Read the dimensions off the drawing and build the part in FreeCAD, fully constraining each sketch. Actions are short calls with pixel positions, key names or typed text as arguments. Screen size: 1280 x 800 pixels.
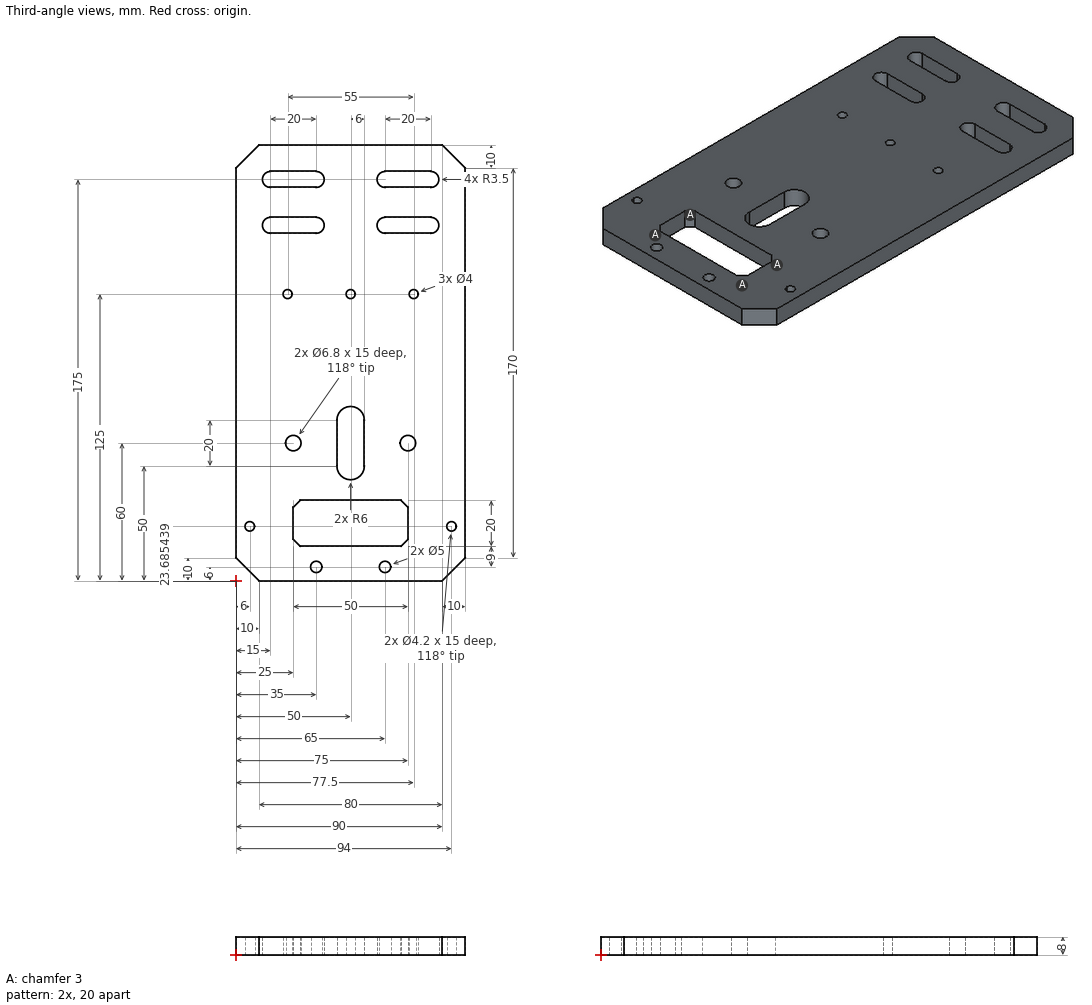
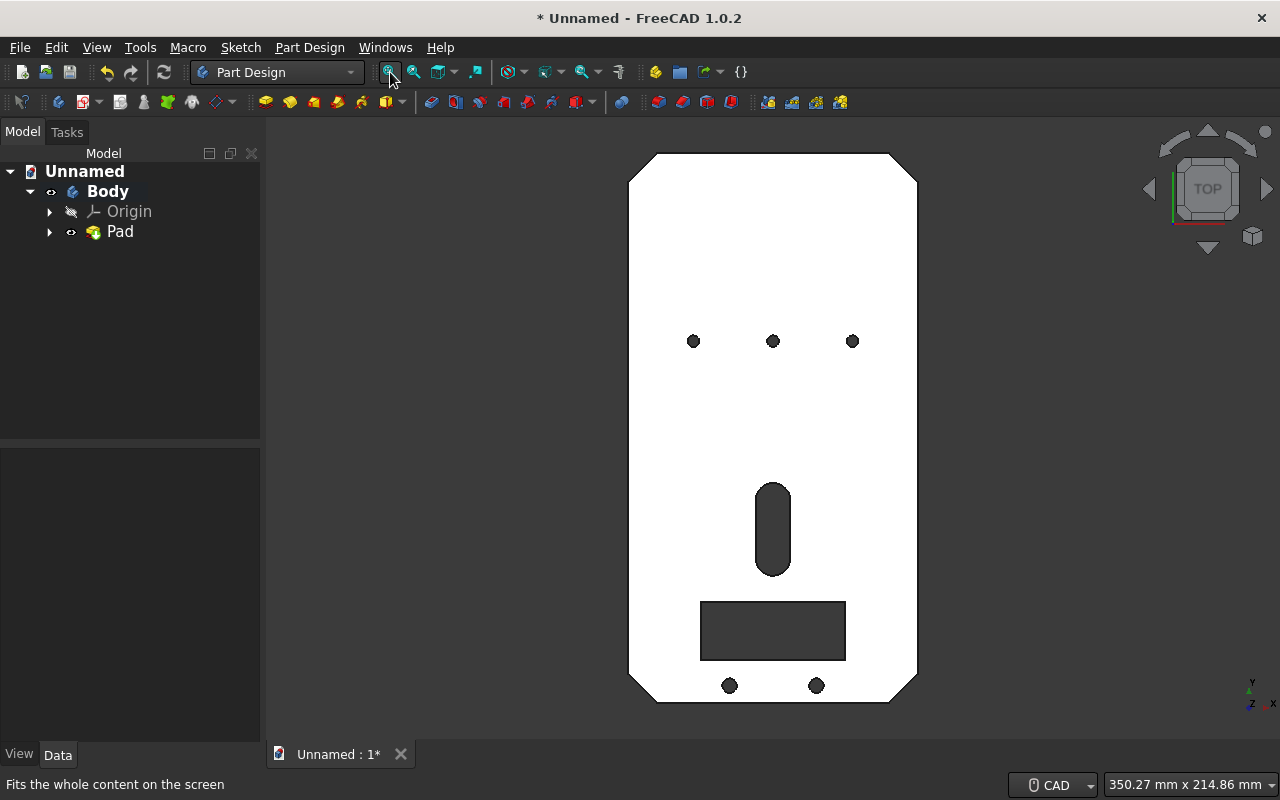
key(1)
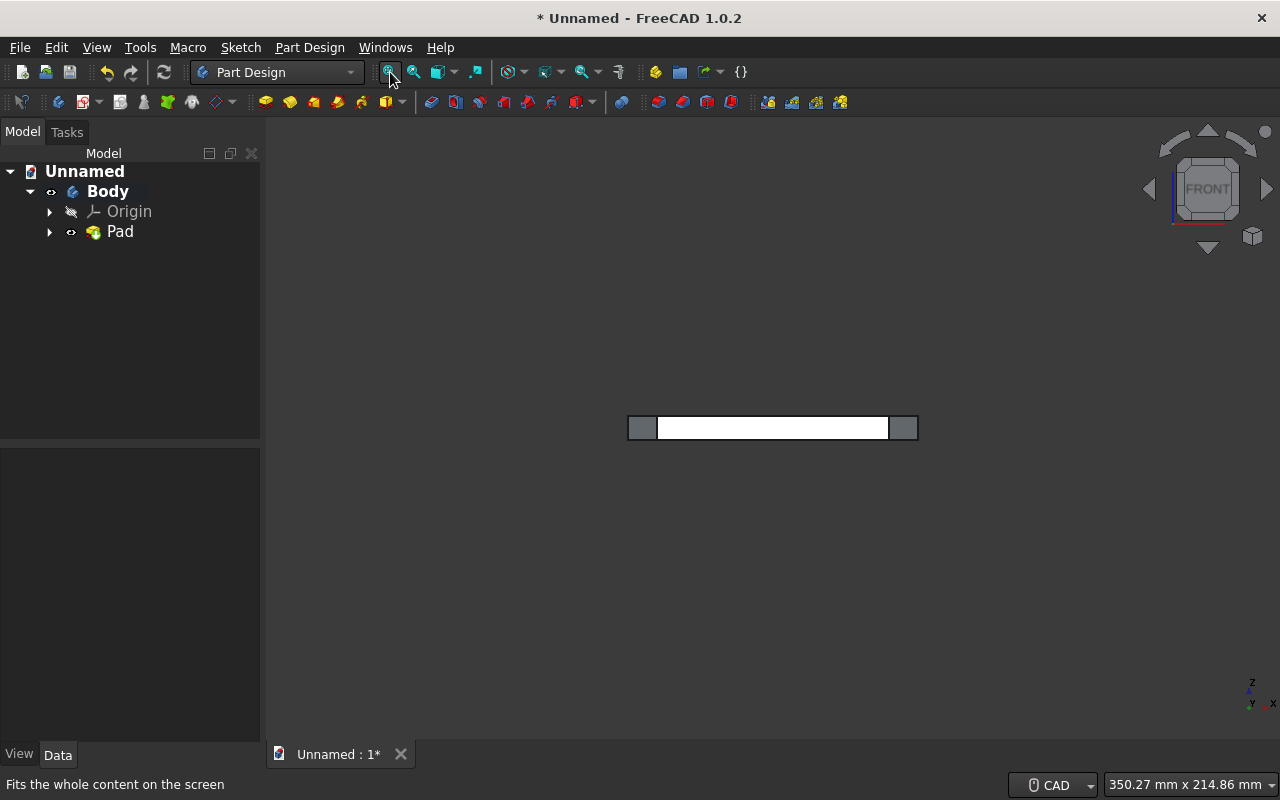
key(v)
key(f)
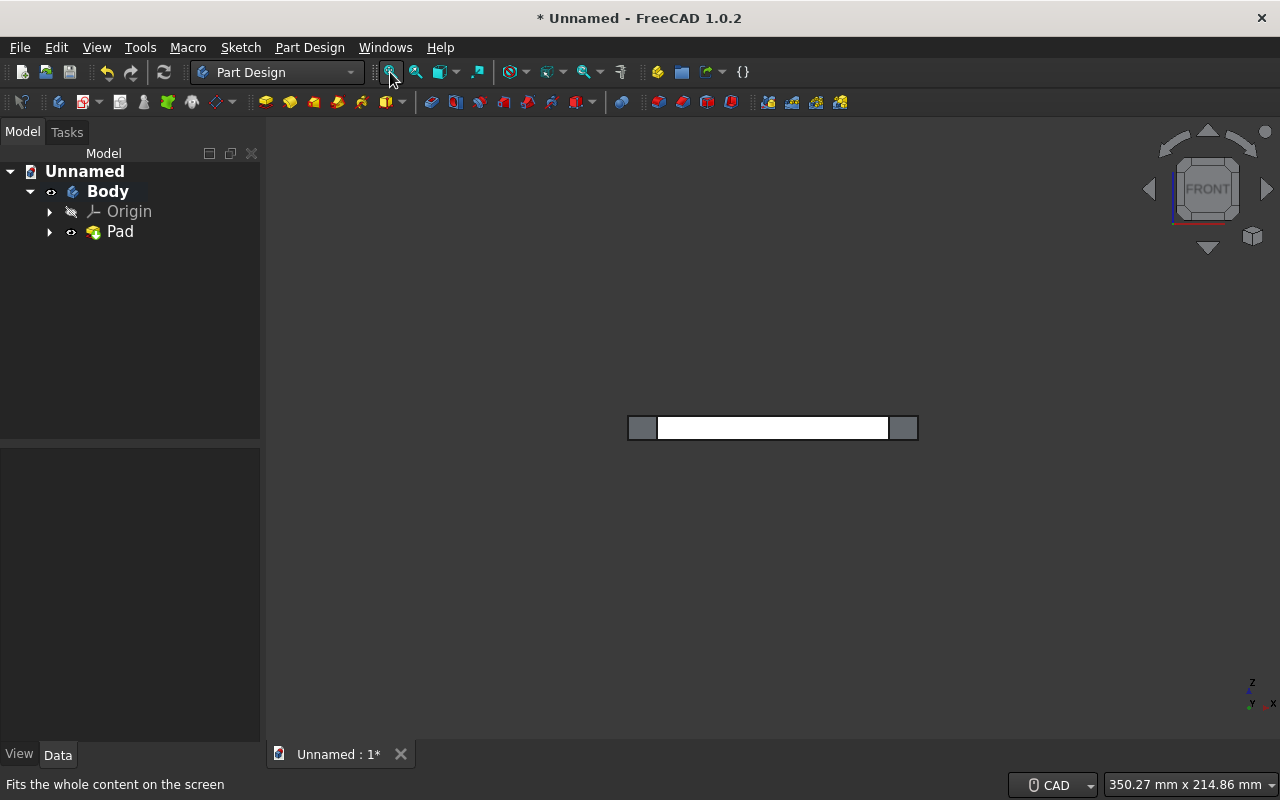
key(3)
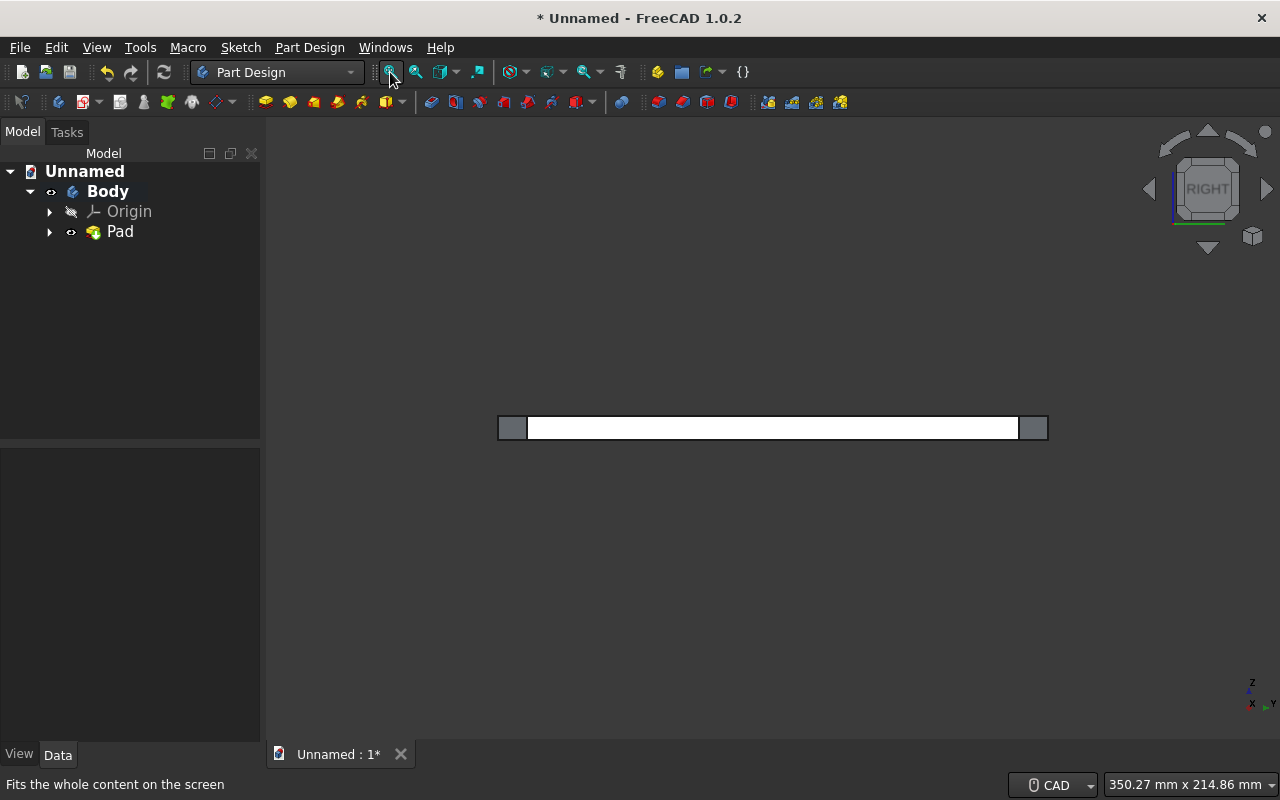
key(5)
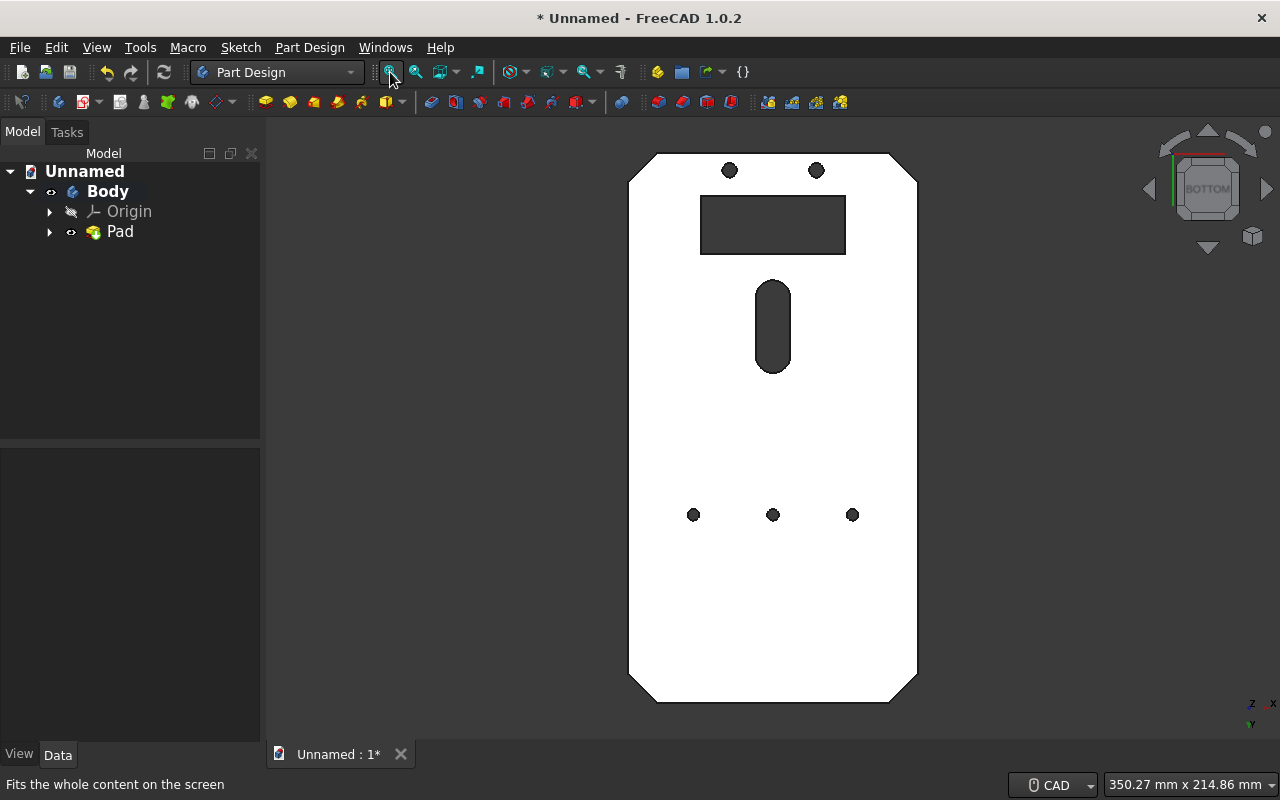
key(4)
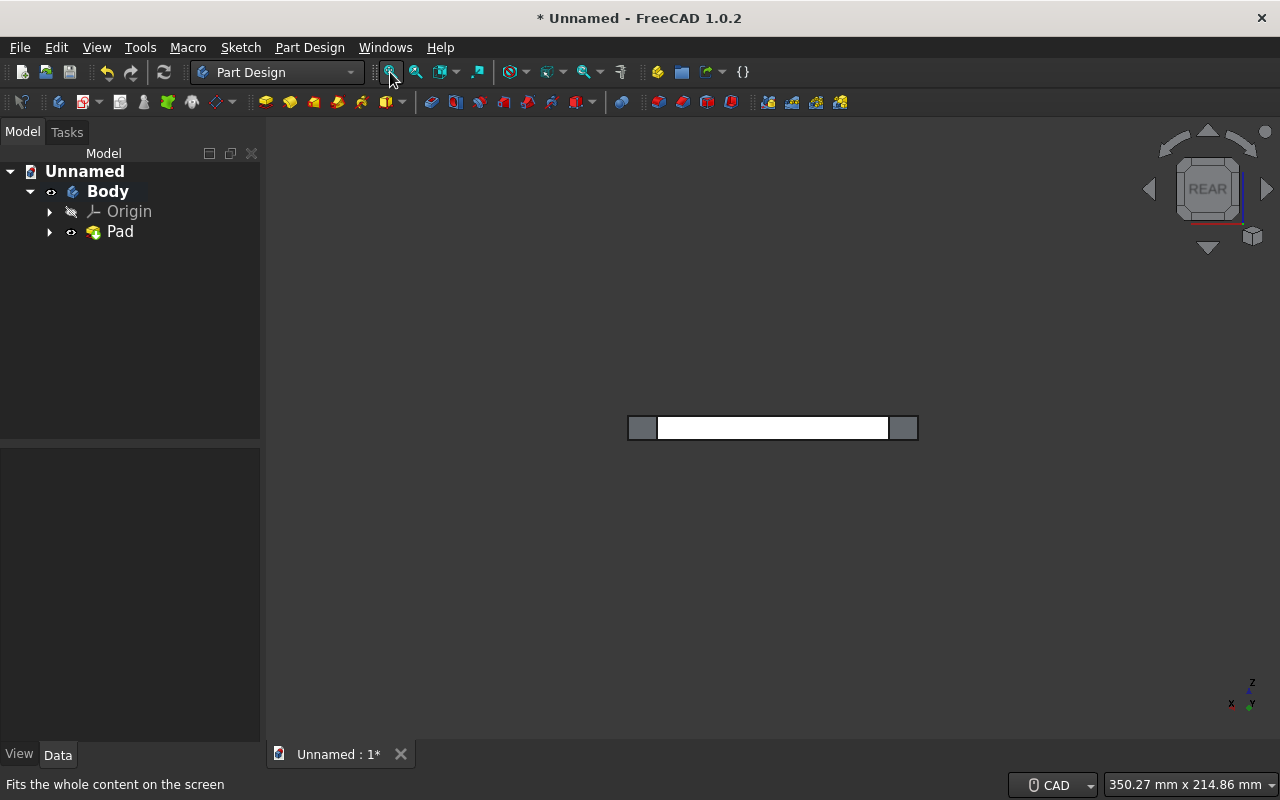
click(392, 72)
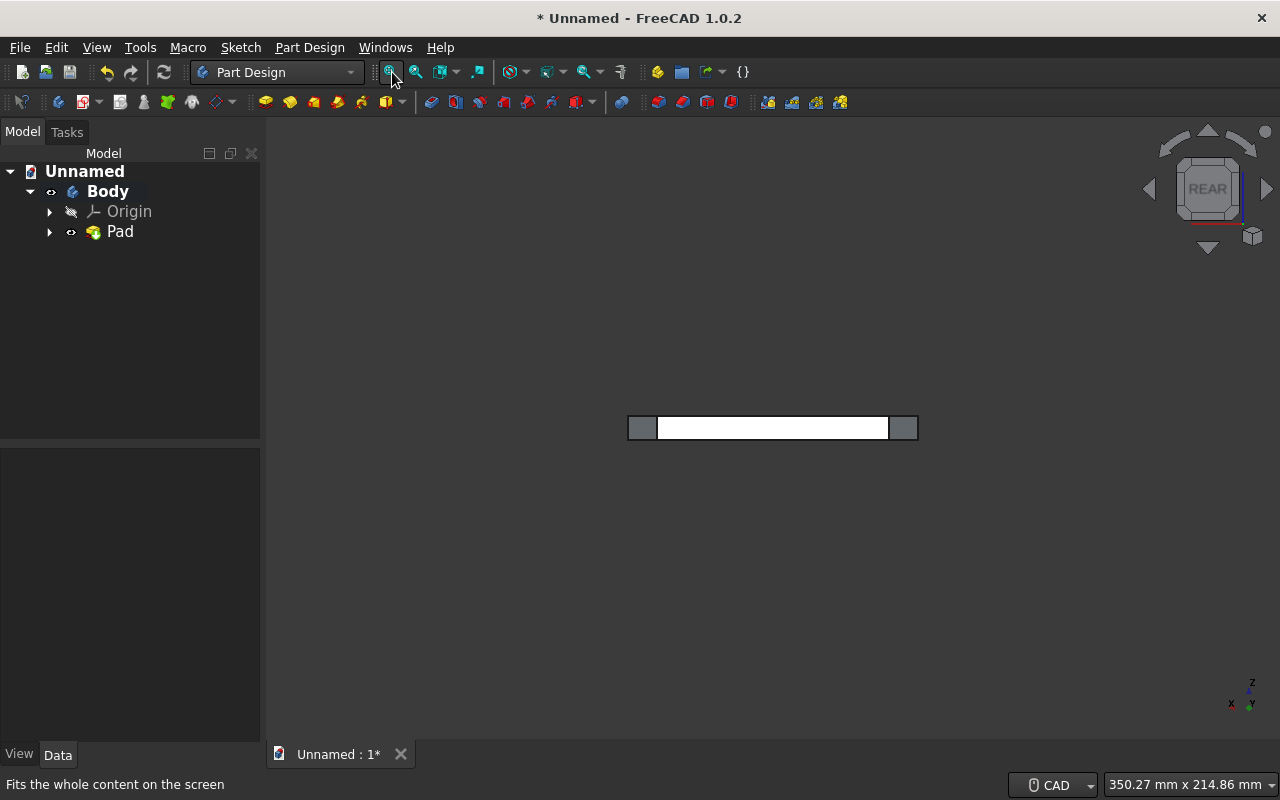
key(6)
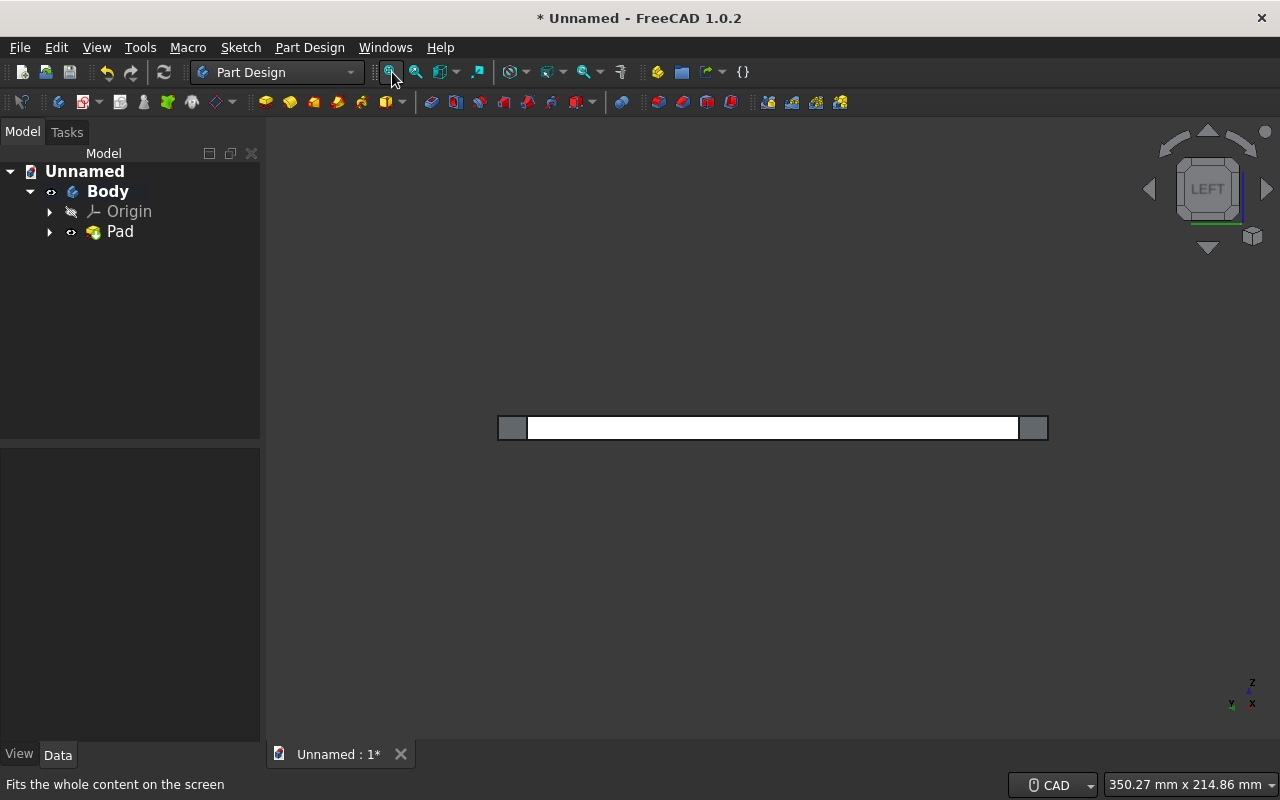
key(v)
key(3)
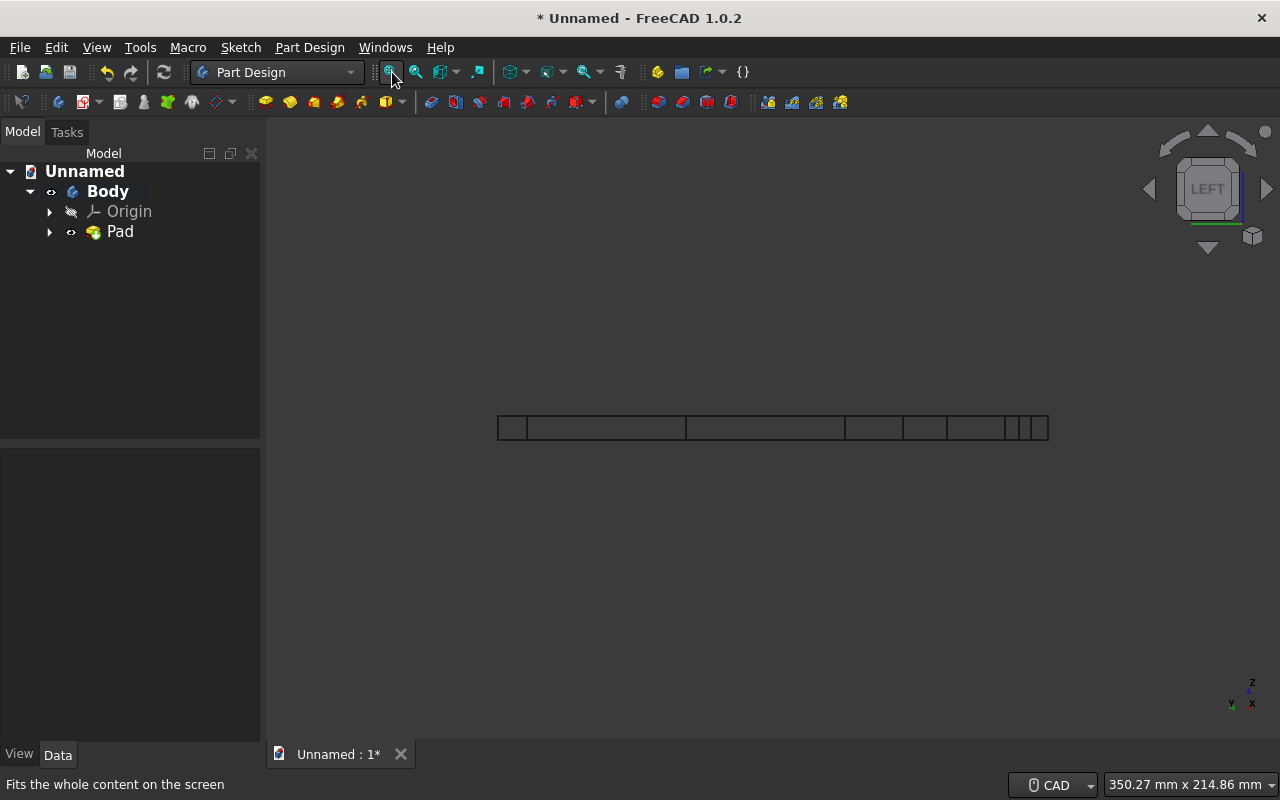
key(0)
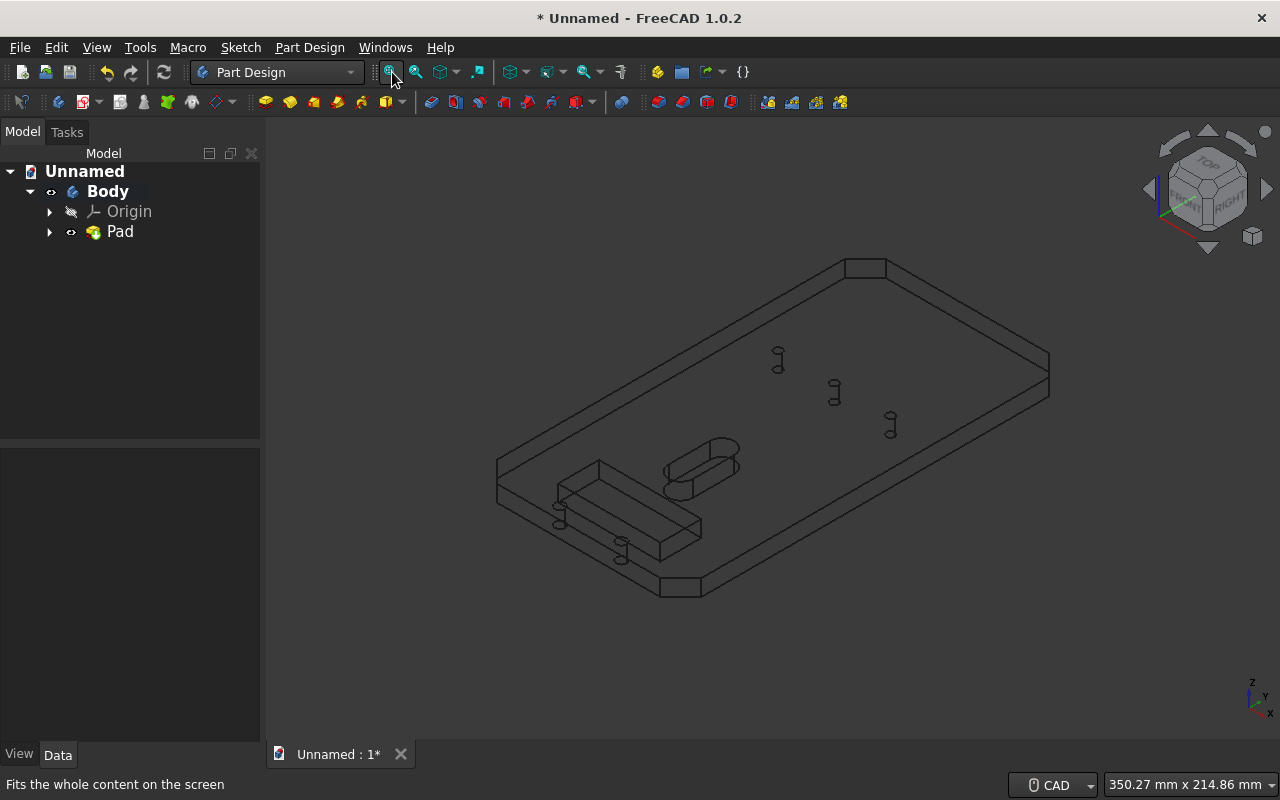
click(599, 468)